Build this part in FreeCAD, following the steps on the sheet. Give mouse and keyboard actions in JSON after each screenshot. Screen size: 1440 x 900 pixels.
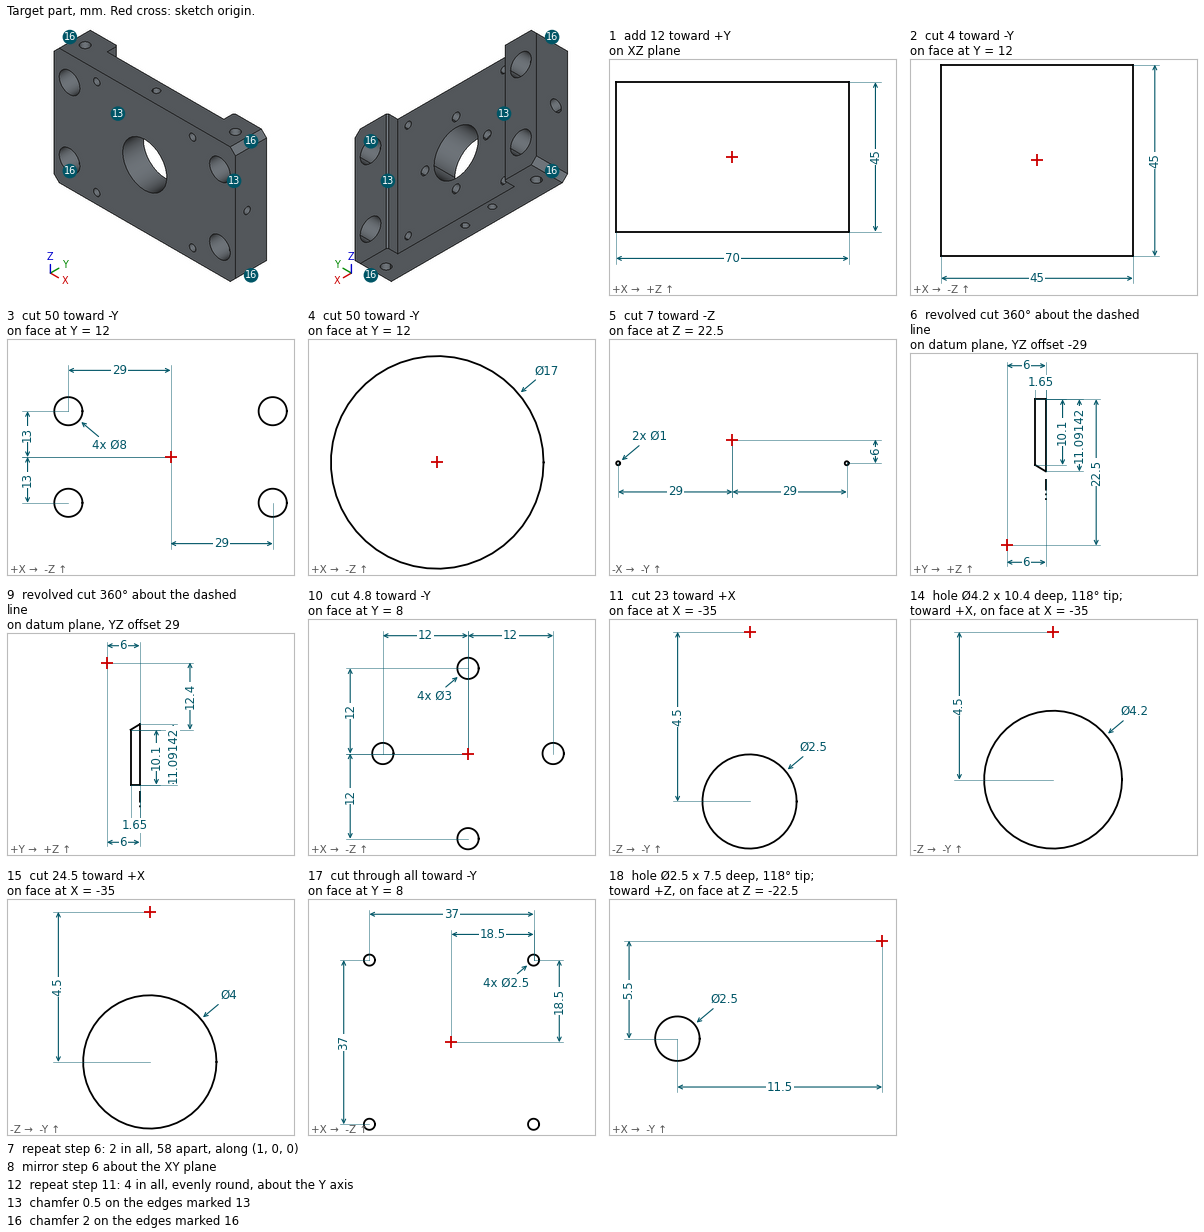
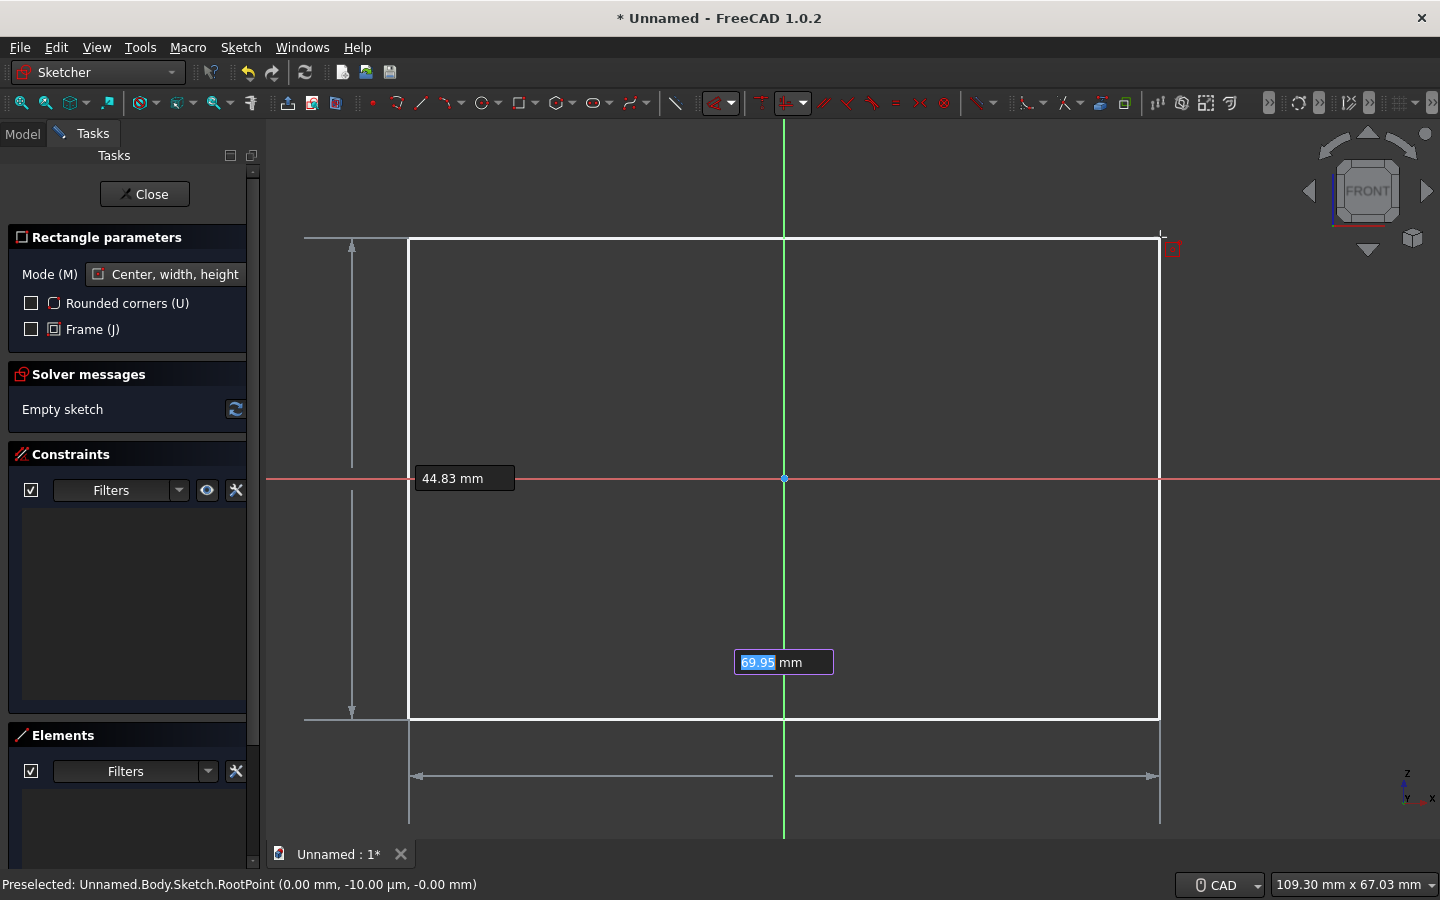
{"action": "type", "text": "70"}
{"action": "key", "text": "Tab"}
{"action": "type", "text": "45"}
{"action": "key", "text": "Return"}
{"action": "key", "text": "Escape"}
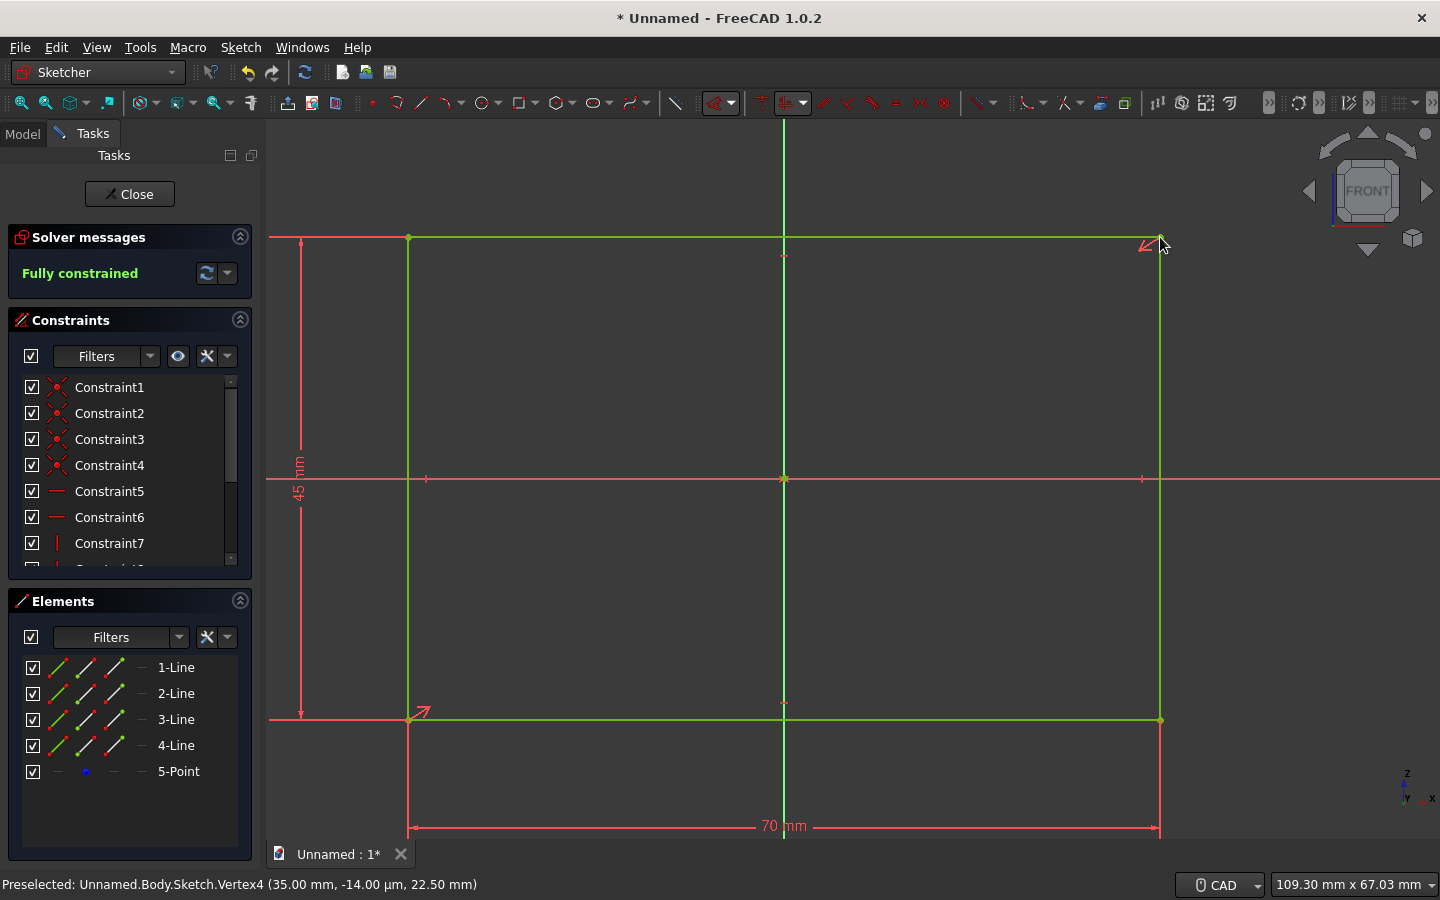
{"action": "left_click", "coordinate": [130, 194]}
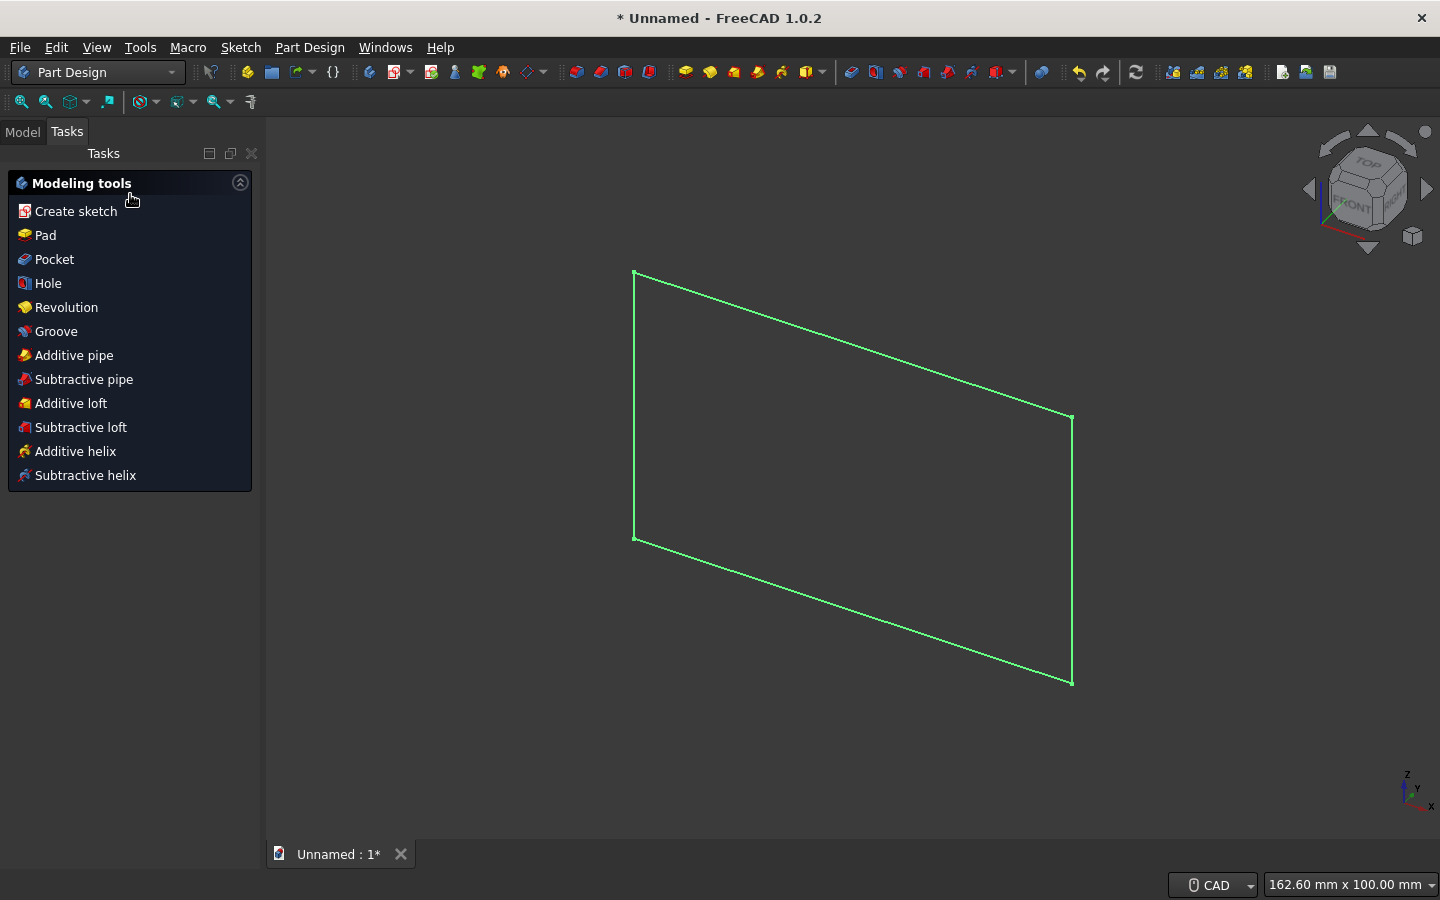
{"action": "left_click", "coordinate": [686, 72]}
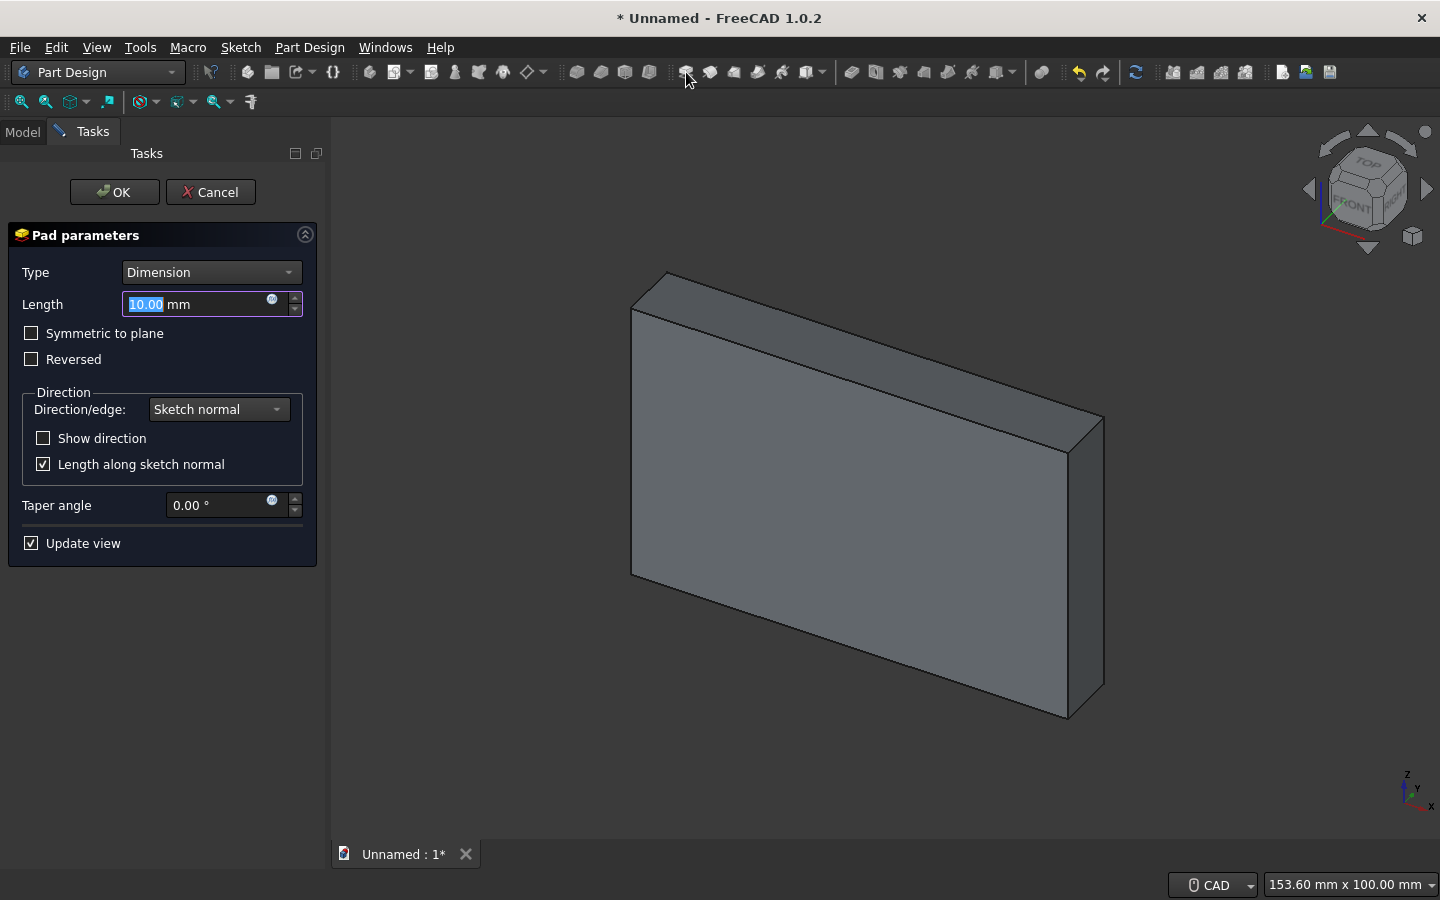
{"action": "type", "text": "12"}
{"action": "key", "text": "Tab"}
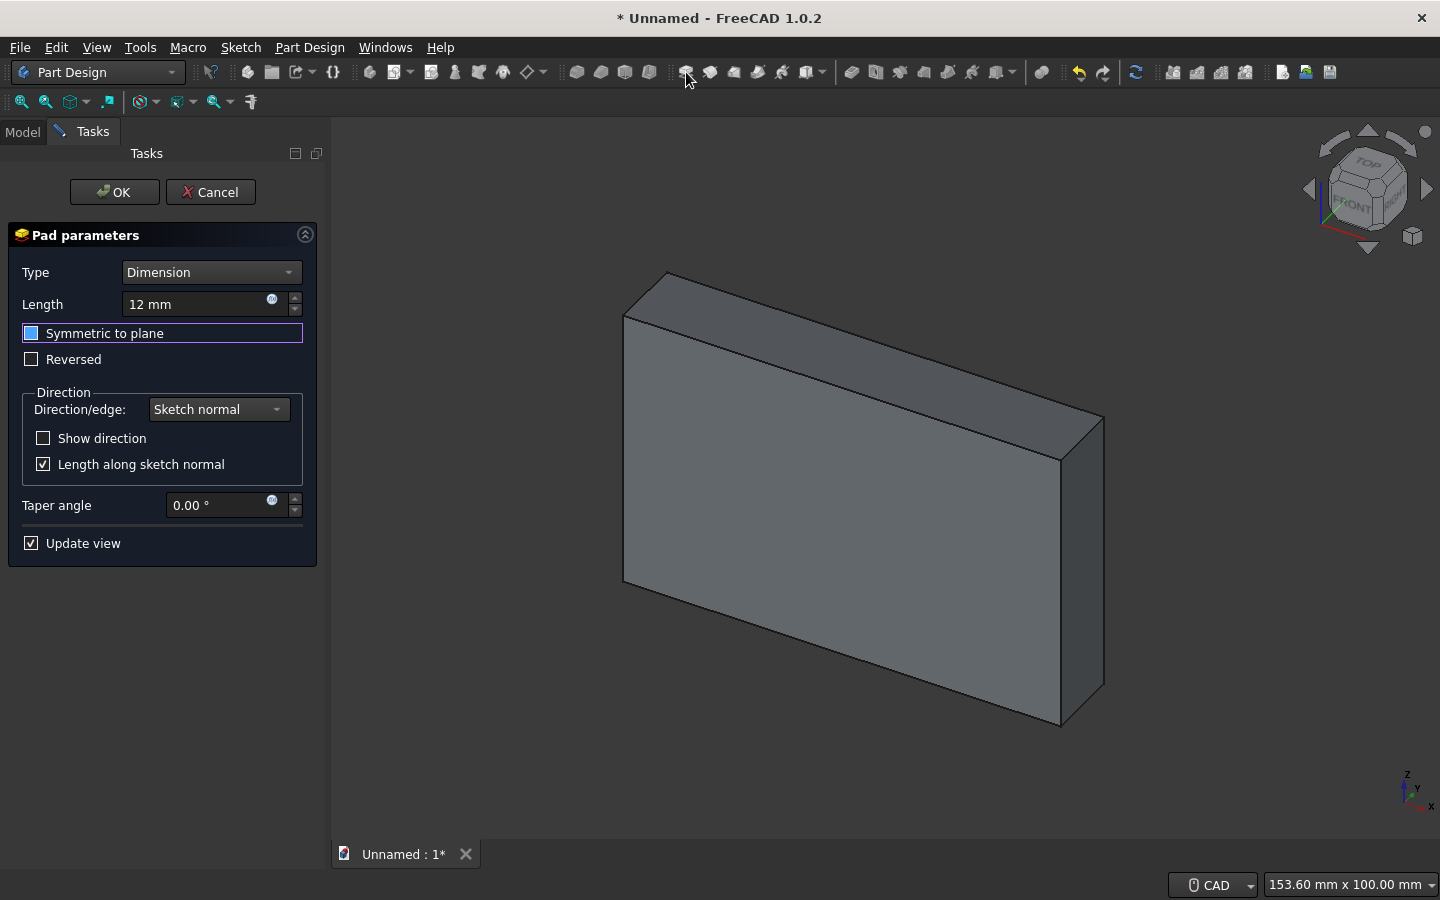
{"action": "left_click", "coordinate": [30, 359]}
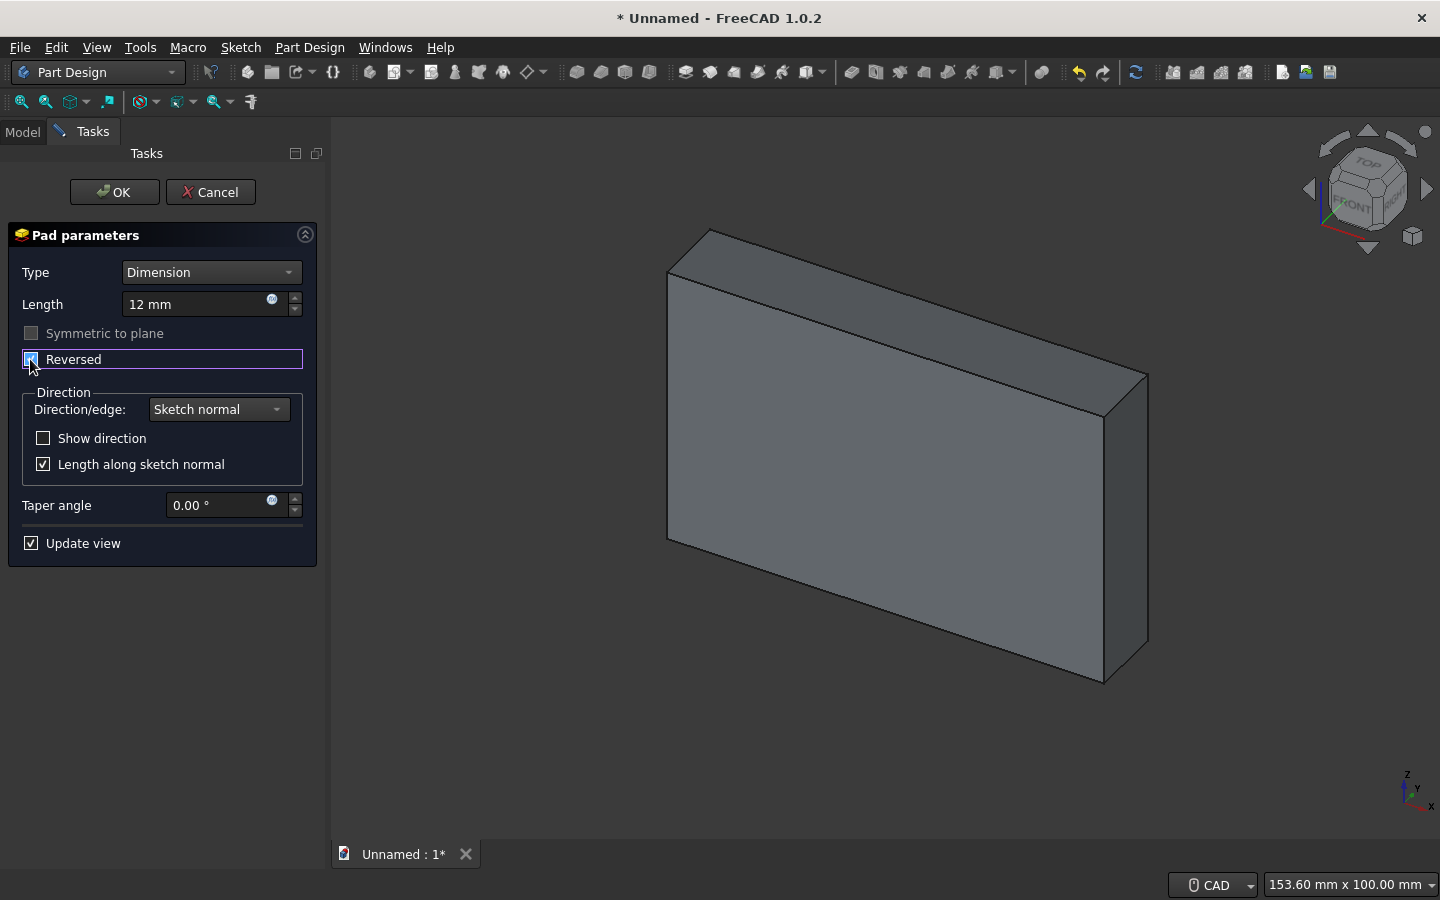
{"action": "left_click", "coordinate": [115, 192]}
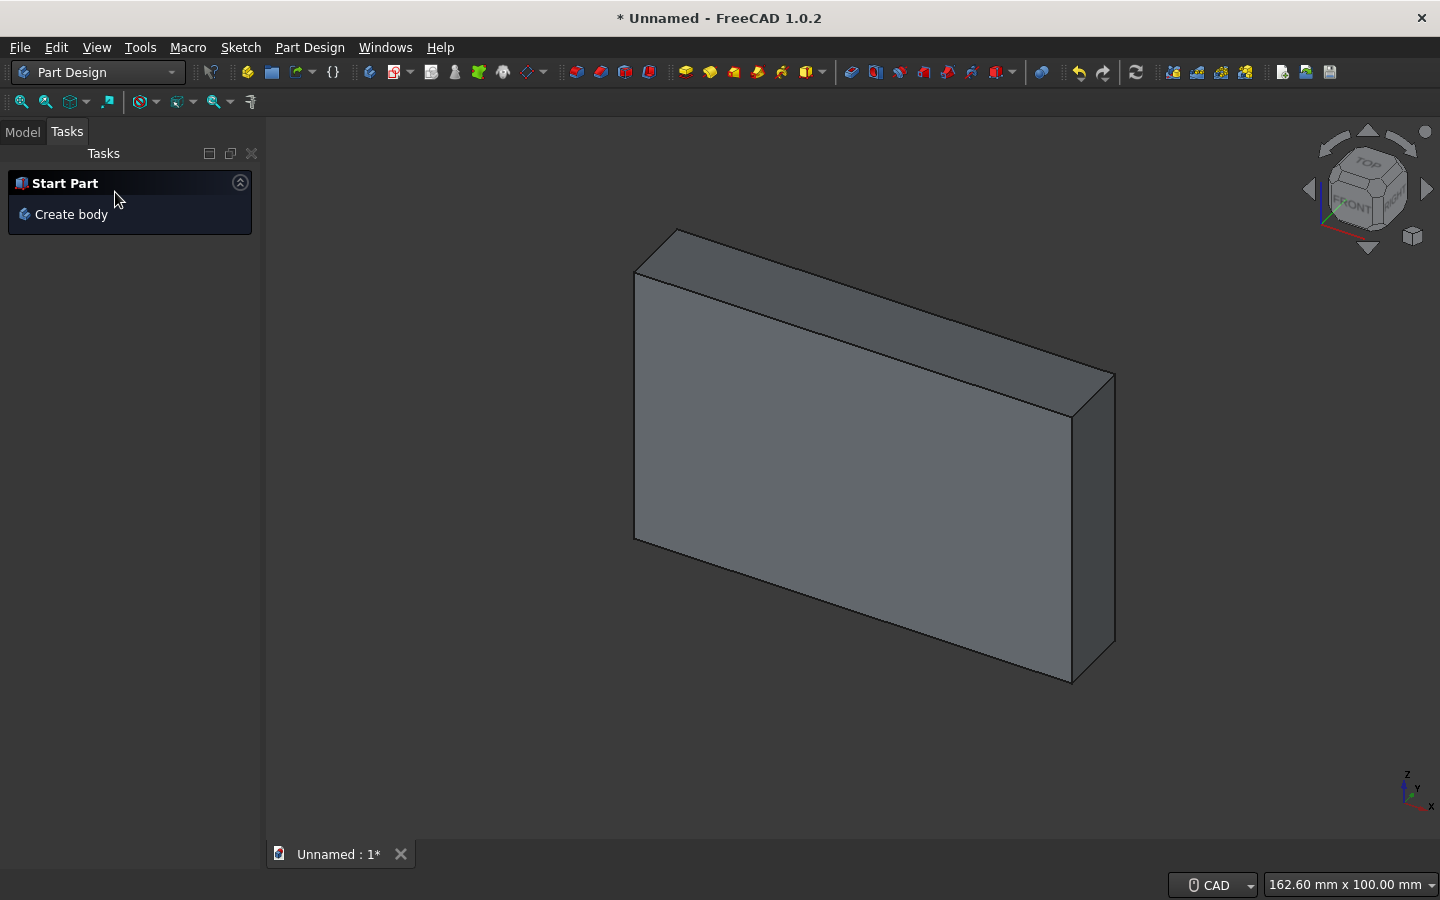
{"action": "key", "text": "4"}